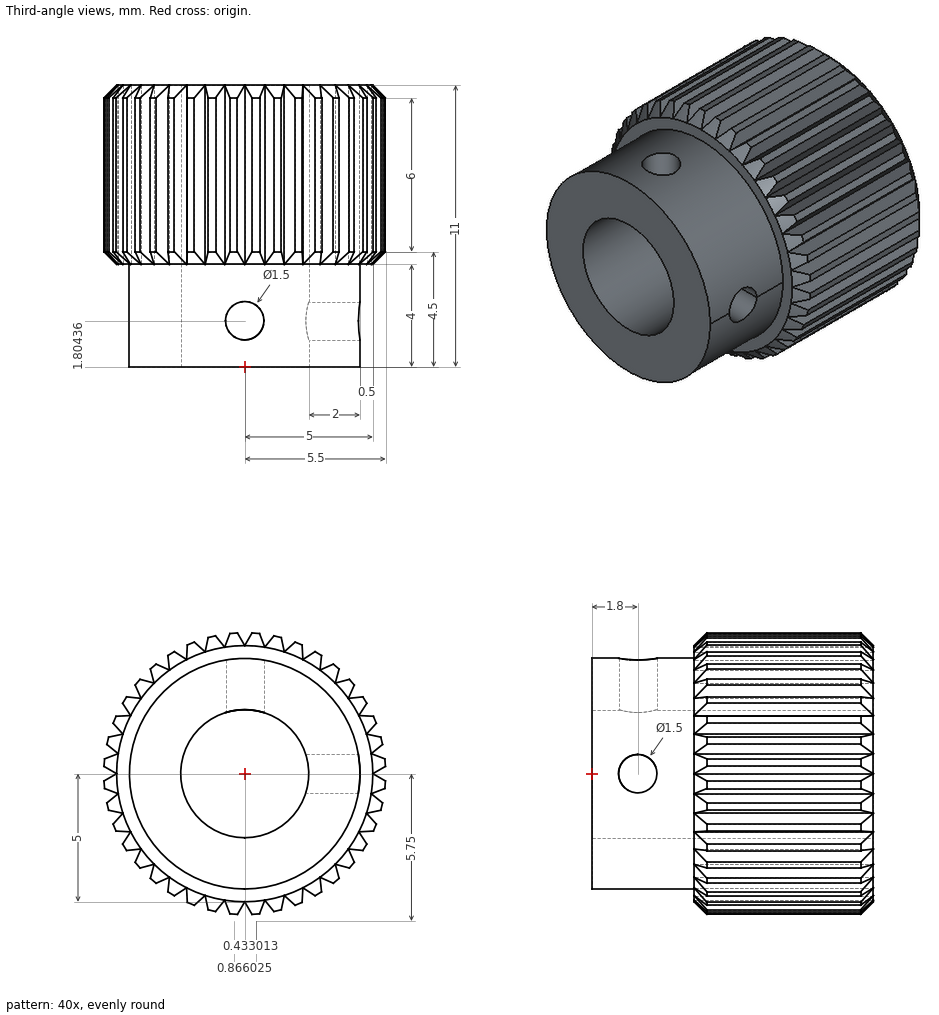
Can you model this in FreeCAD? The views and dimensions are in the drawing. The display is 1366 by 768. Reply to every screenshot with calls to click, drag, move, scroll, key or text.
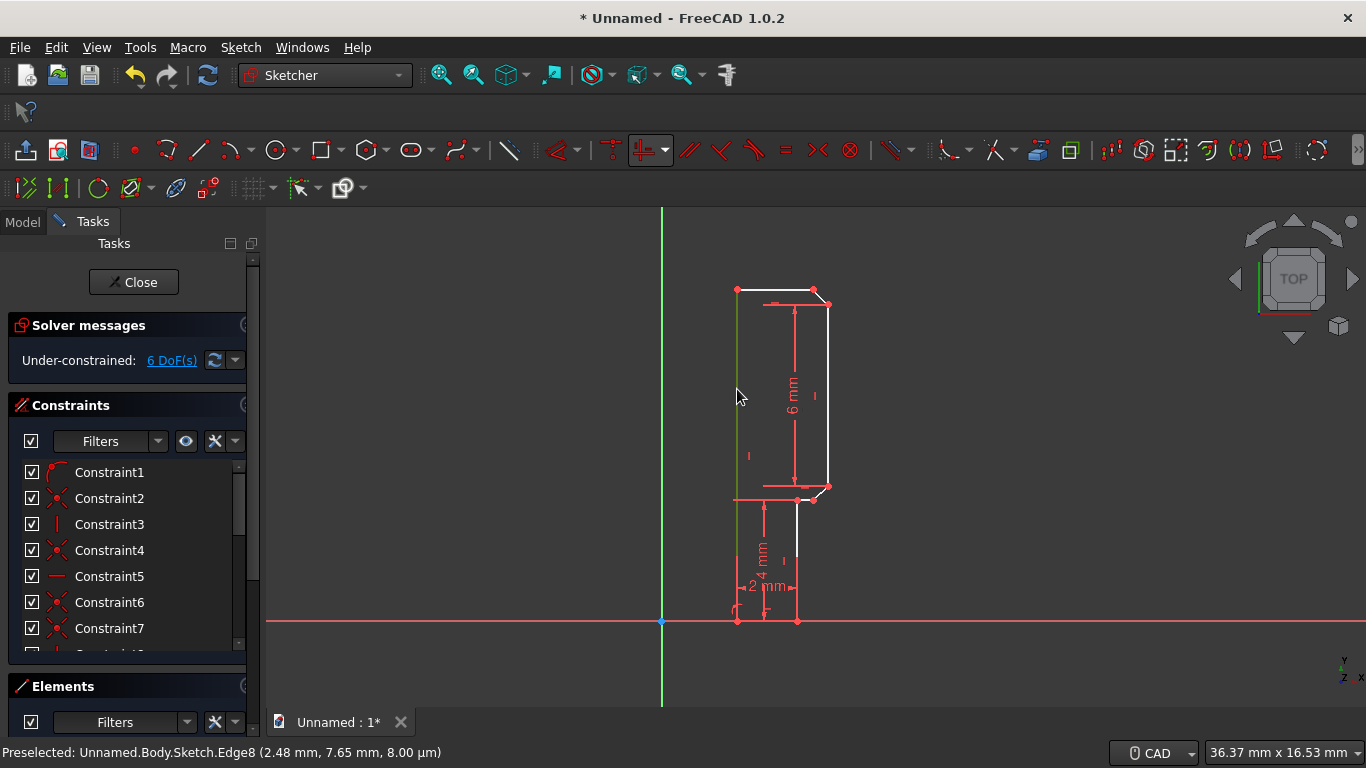
key(i)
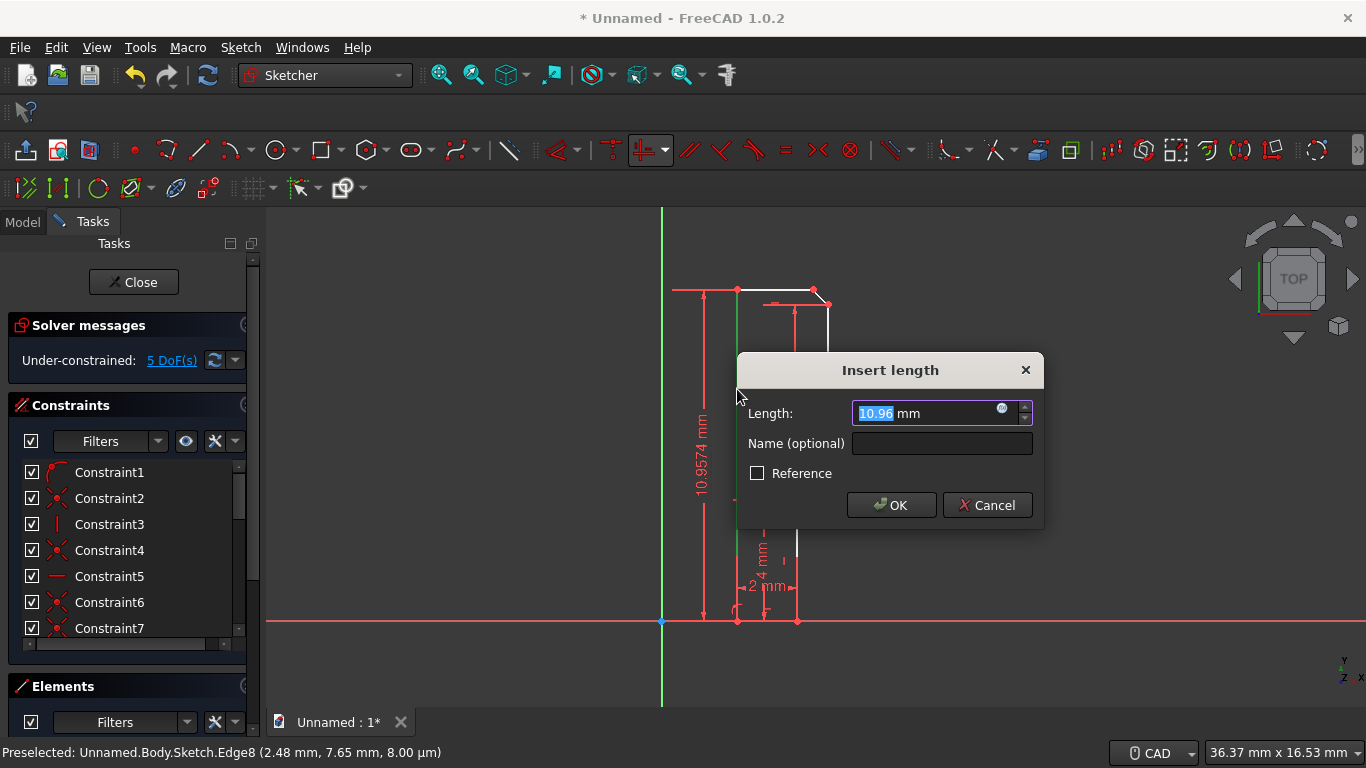
text(11)
key(Return)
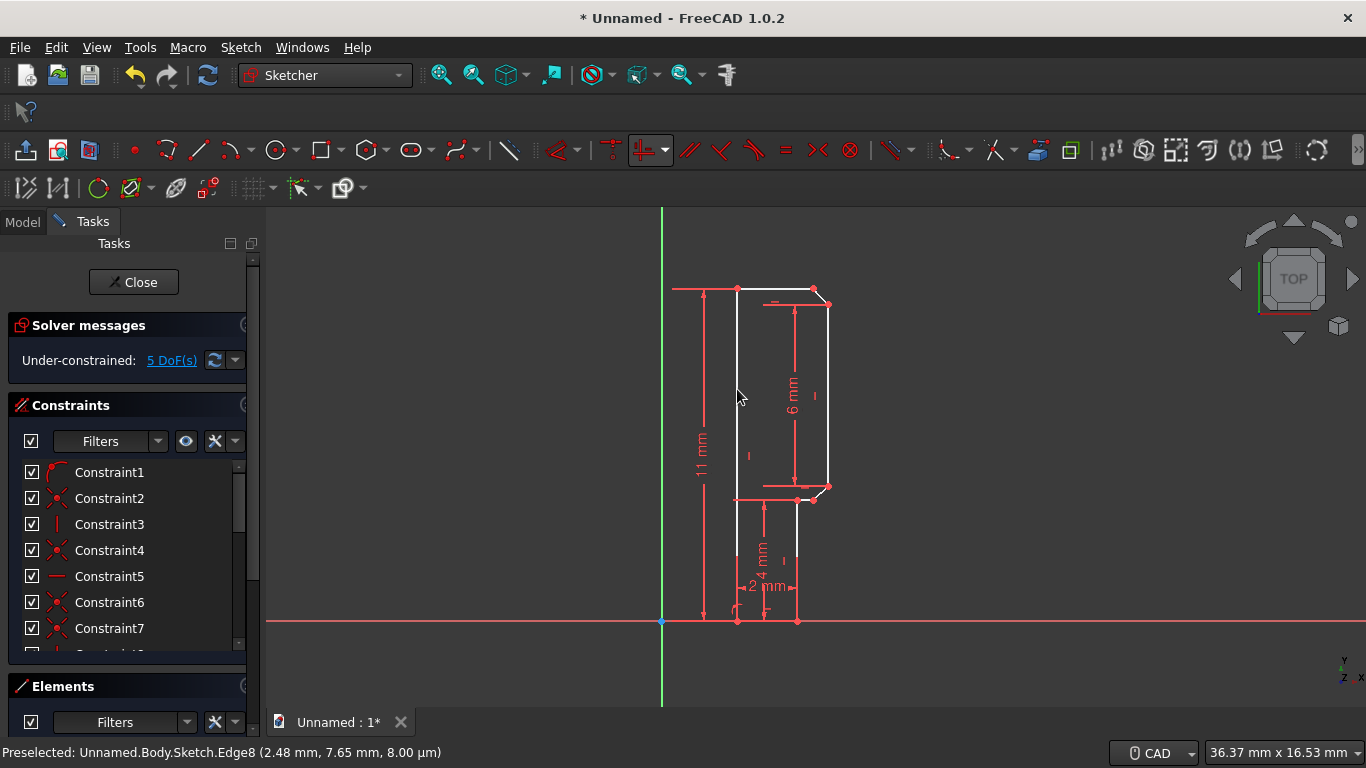
click(813, 500)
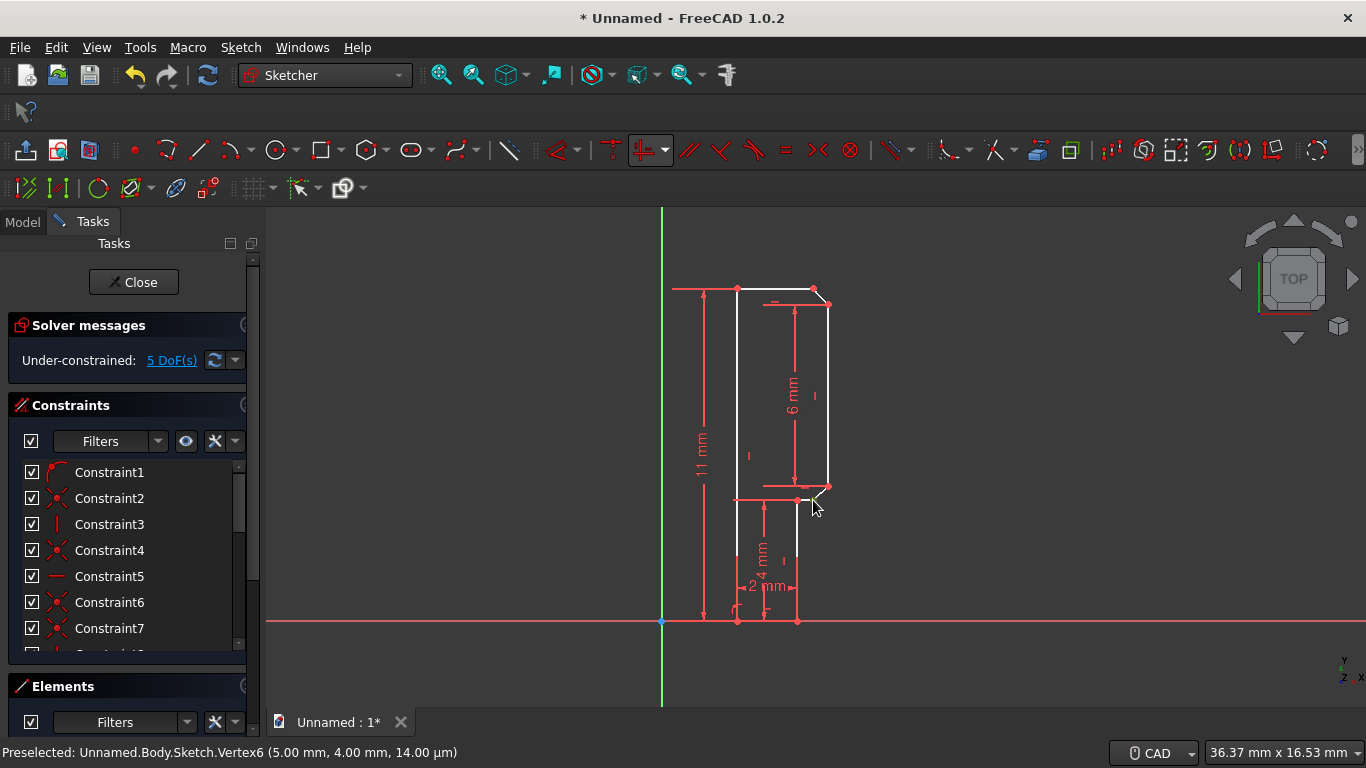
click(580, 150)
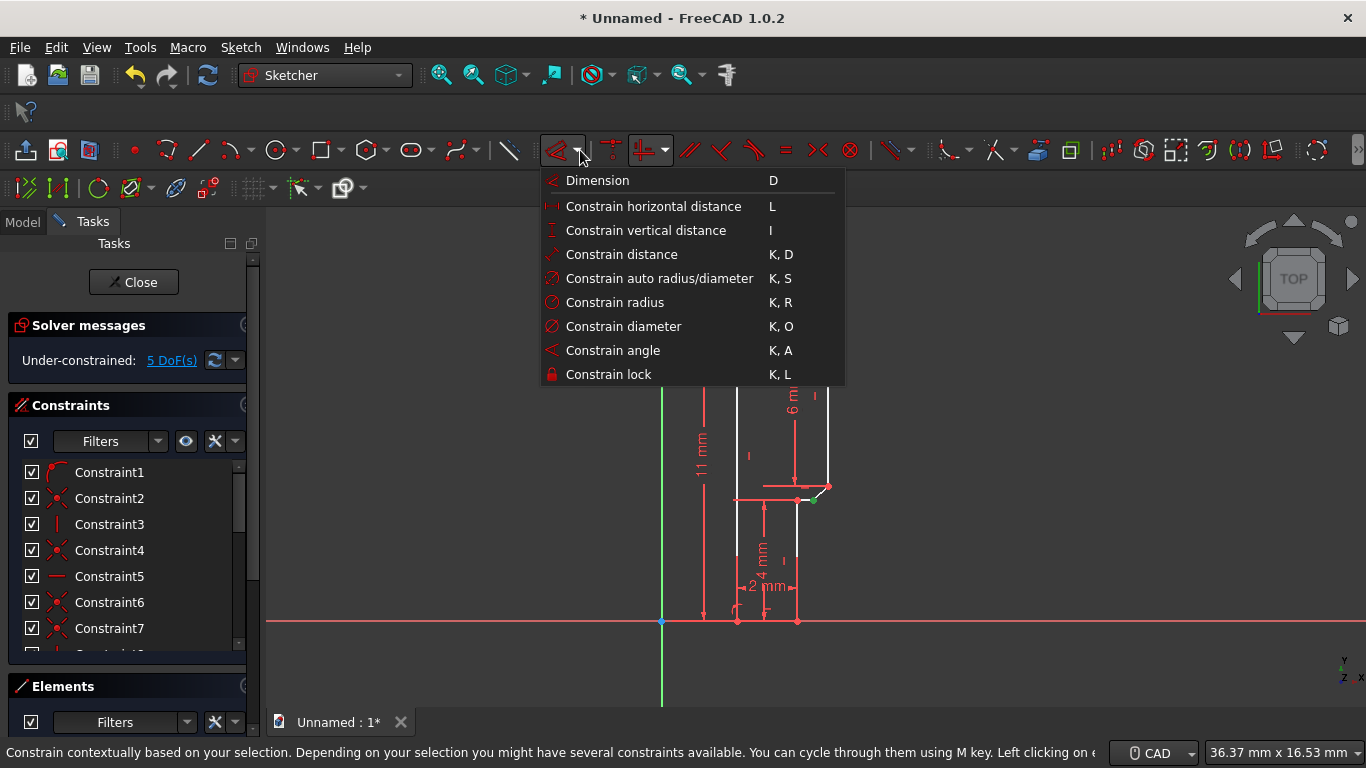
click(693, 206)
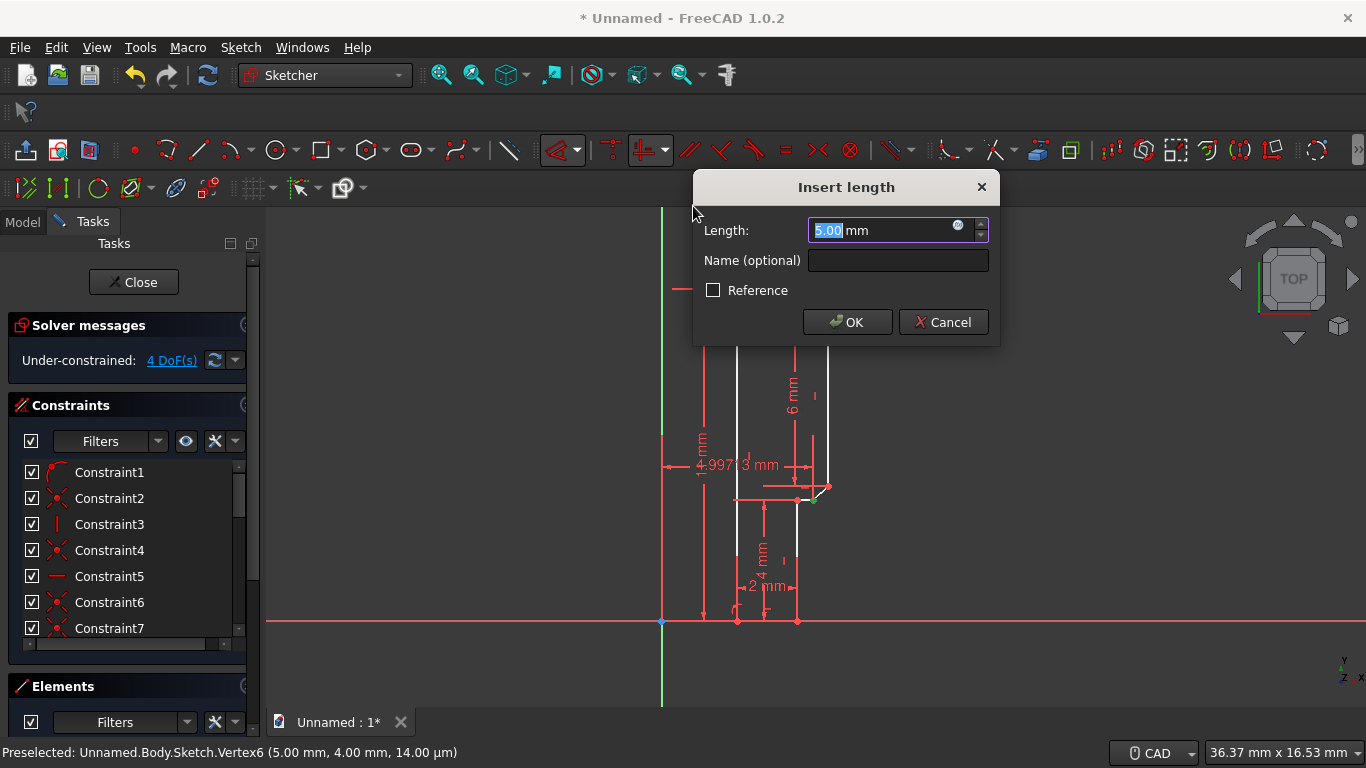
text(5)
key(Return)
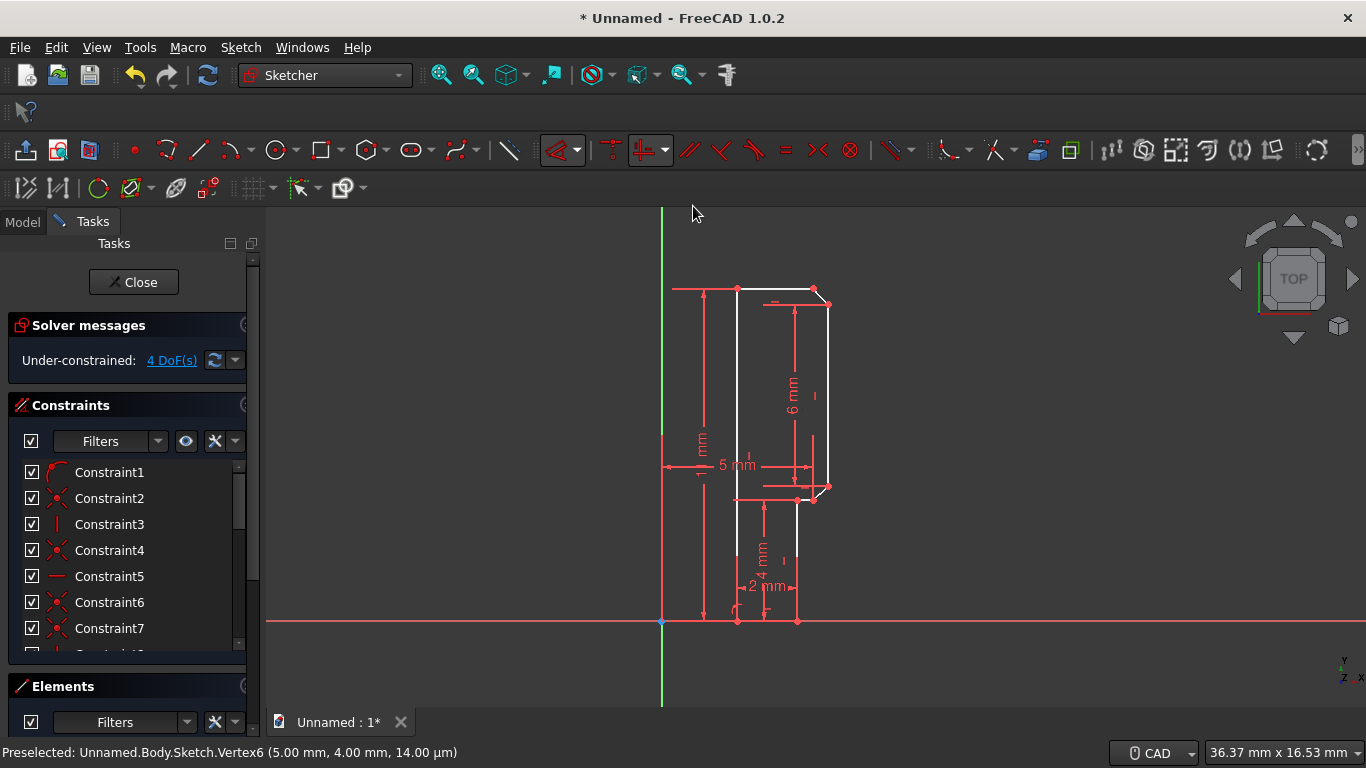
click(813, 289)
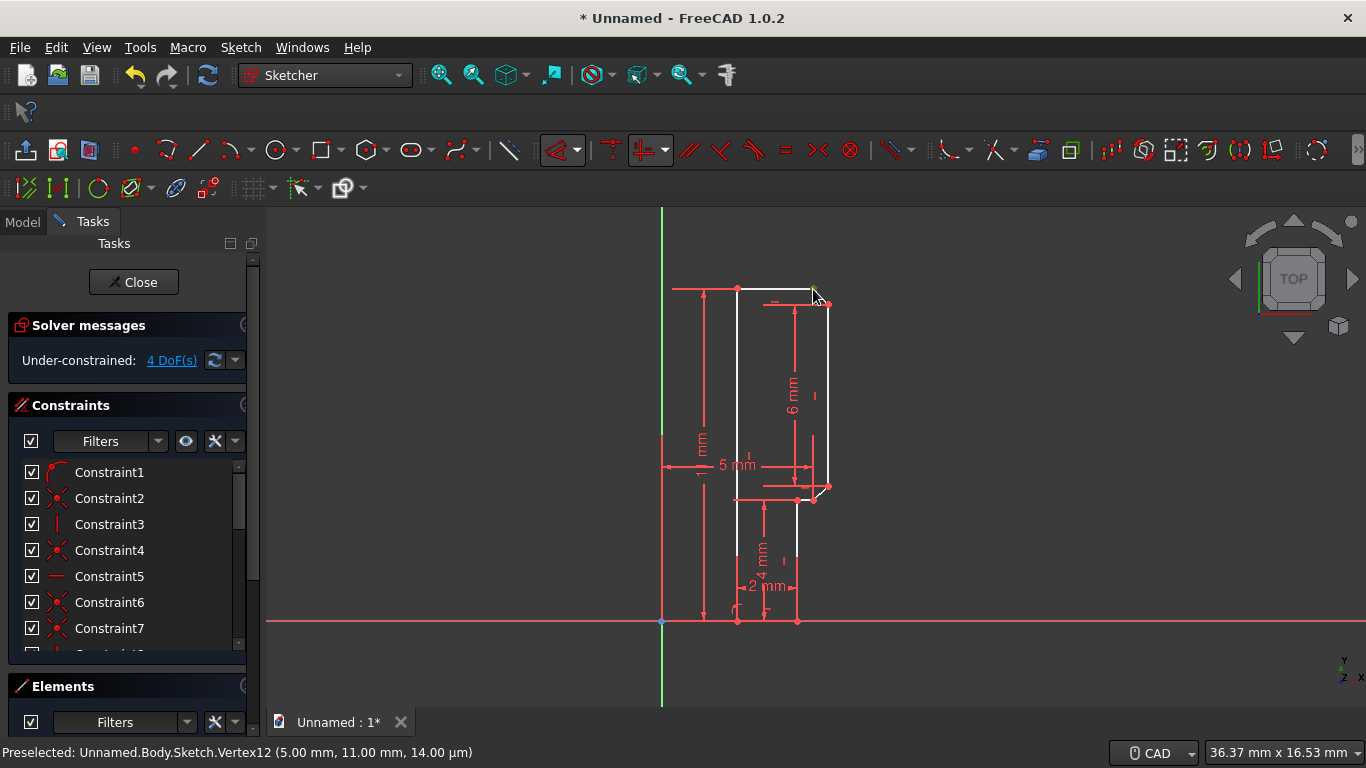
key(l)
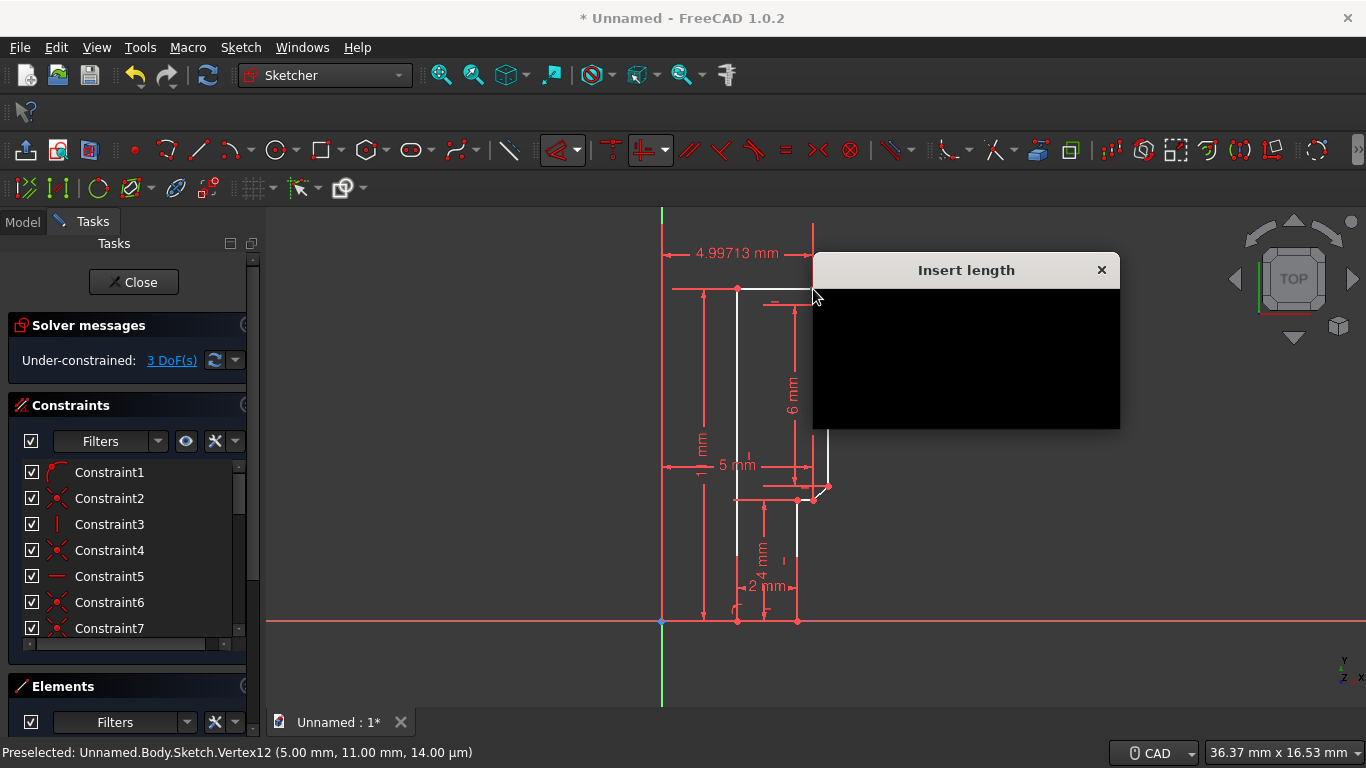
text(5)
key(Return)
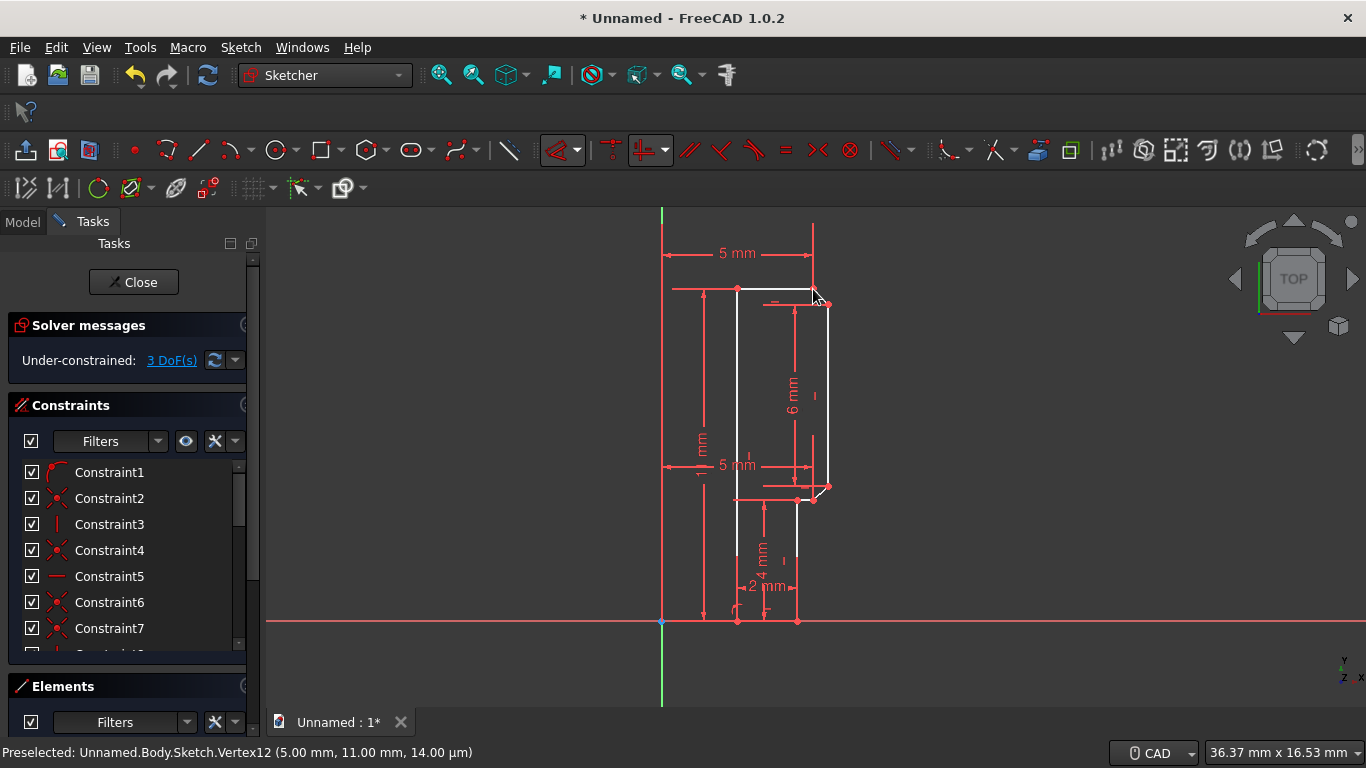
scroll(805, 500, up, 5)